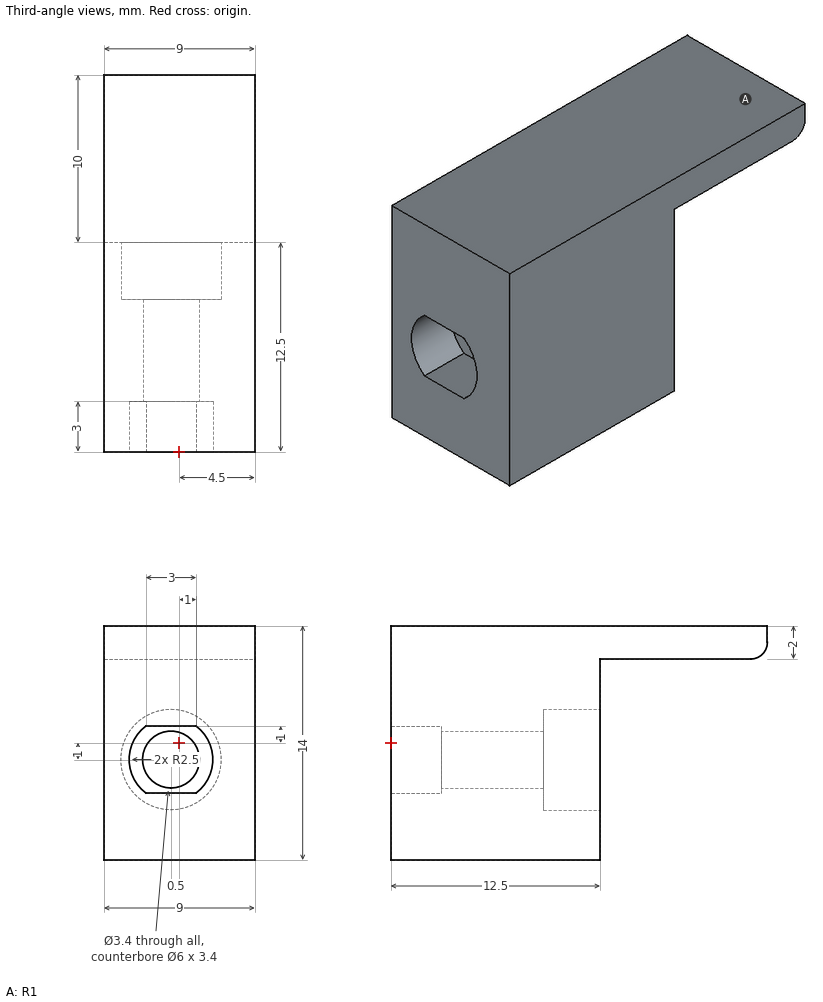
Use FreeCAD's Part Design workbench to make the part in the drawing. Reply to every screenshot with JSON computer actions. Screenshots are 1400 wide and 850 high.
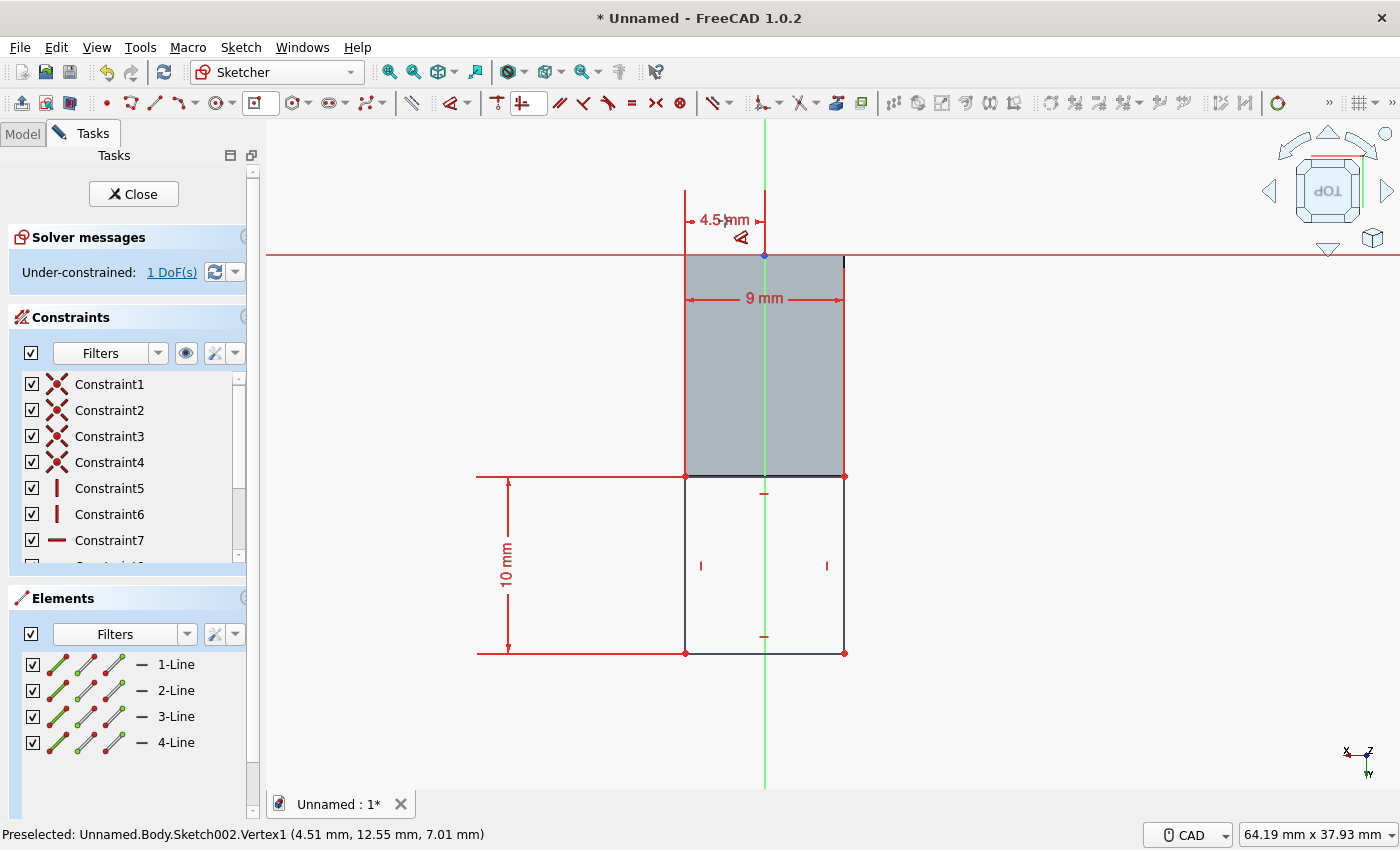
{"action": "left_click", "coordinate": [685, 477]}
{"action": "left_click", "coordinate": [651, 366]}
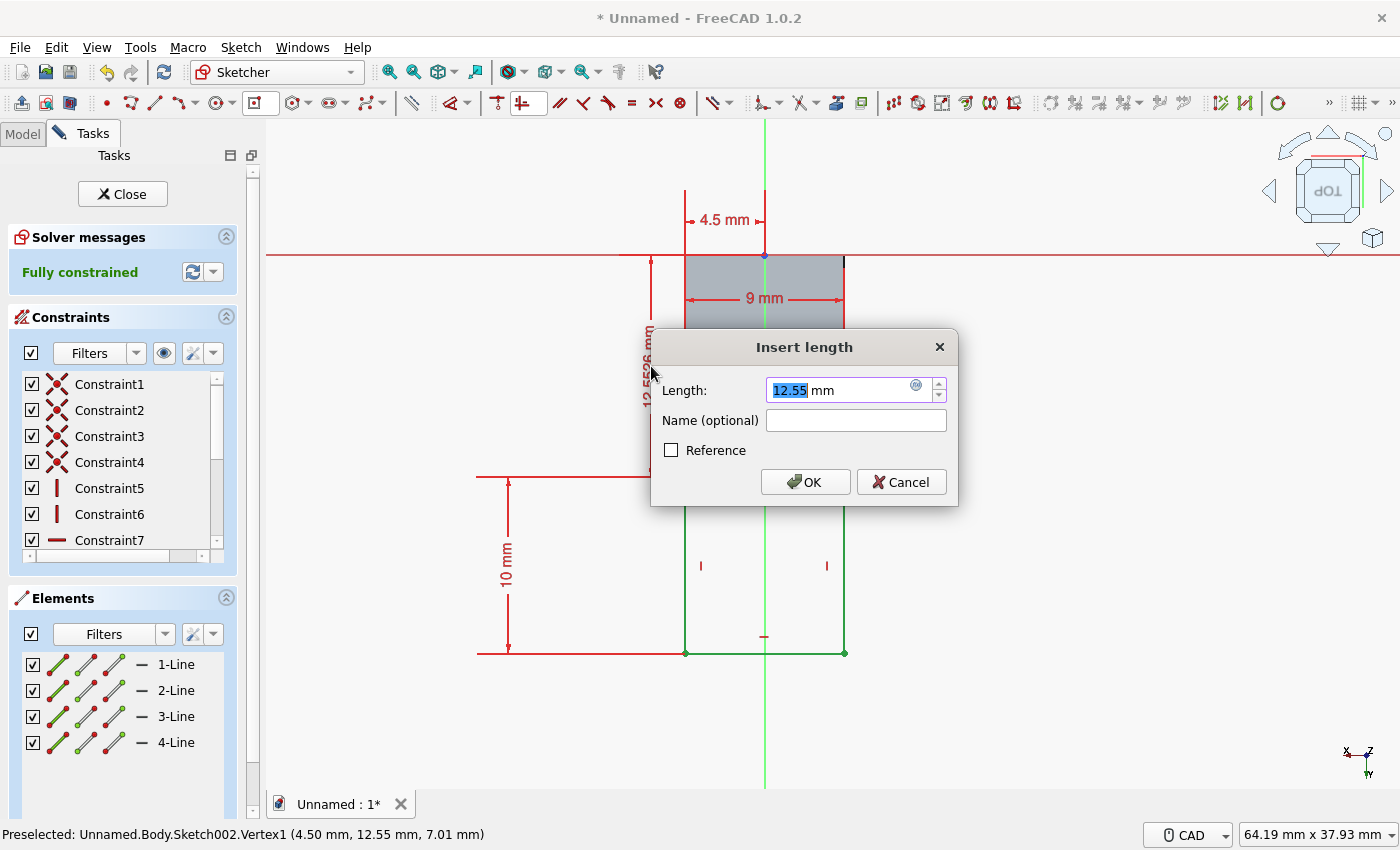
{"action": "type", "text": "12.5"}
{"action": "key", "text": "Return"}
{"action": "key", "text": "Escape"}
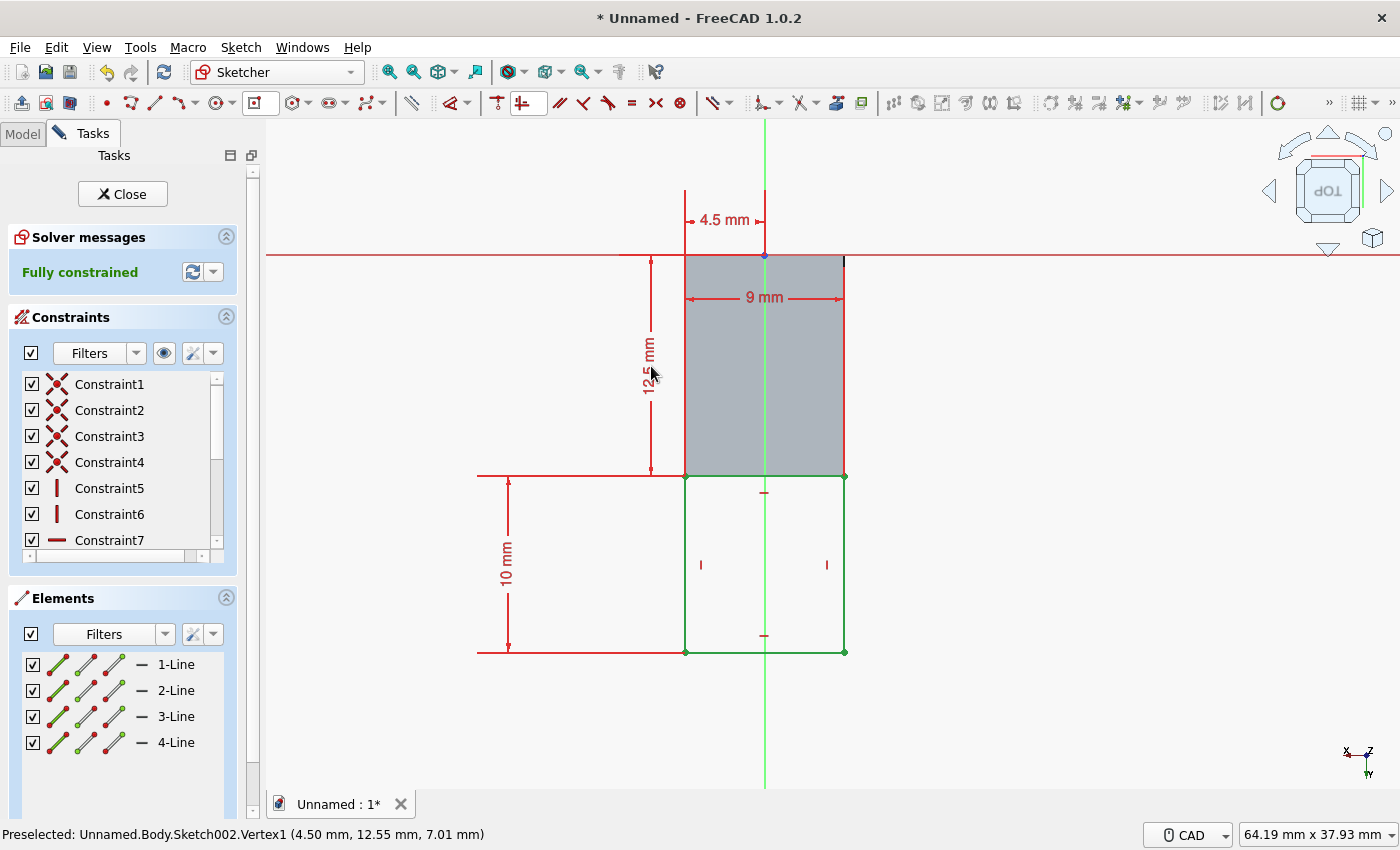
{"action": "left_click", "coordinate": [123, 194]}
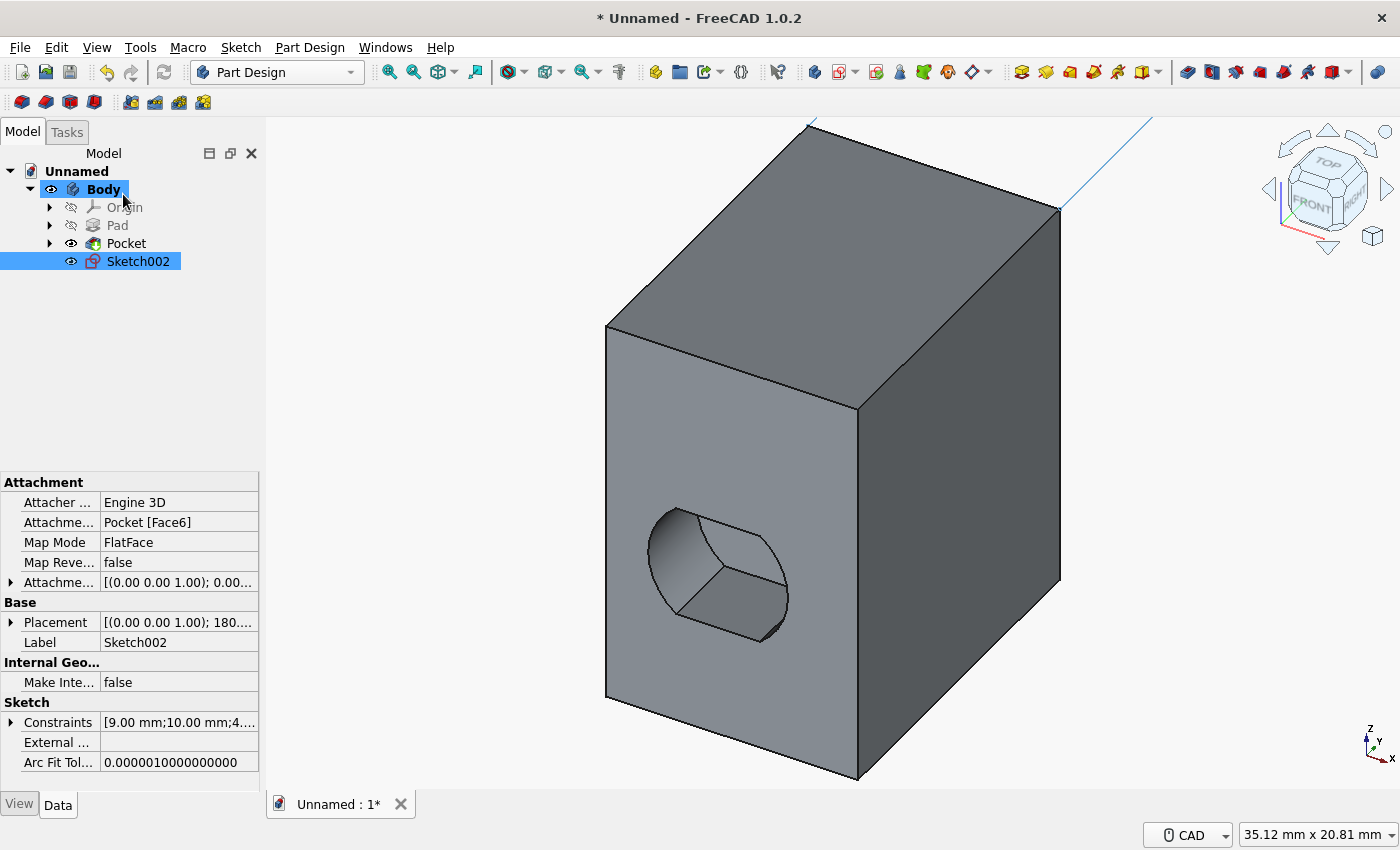
{"action": "left_click", "coordinate": [1022, 72]}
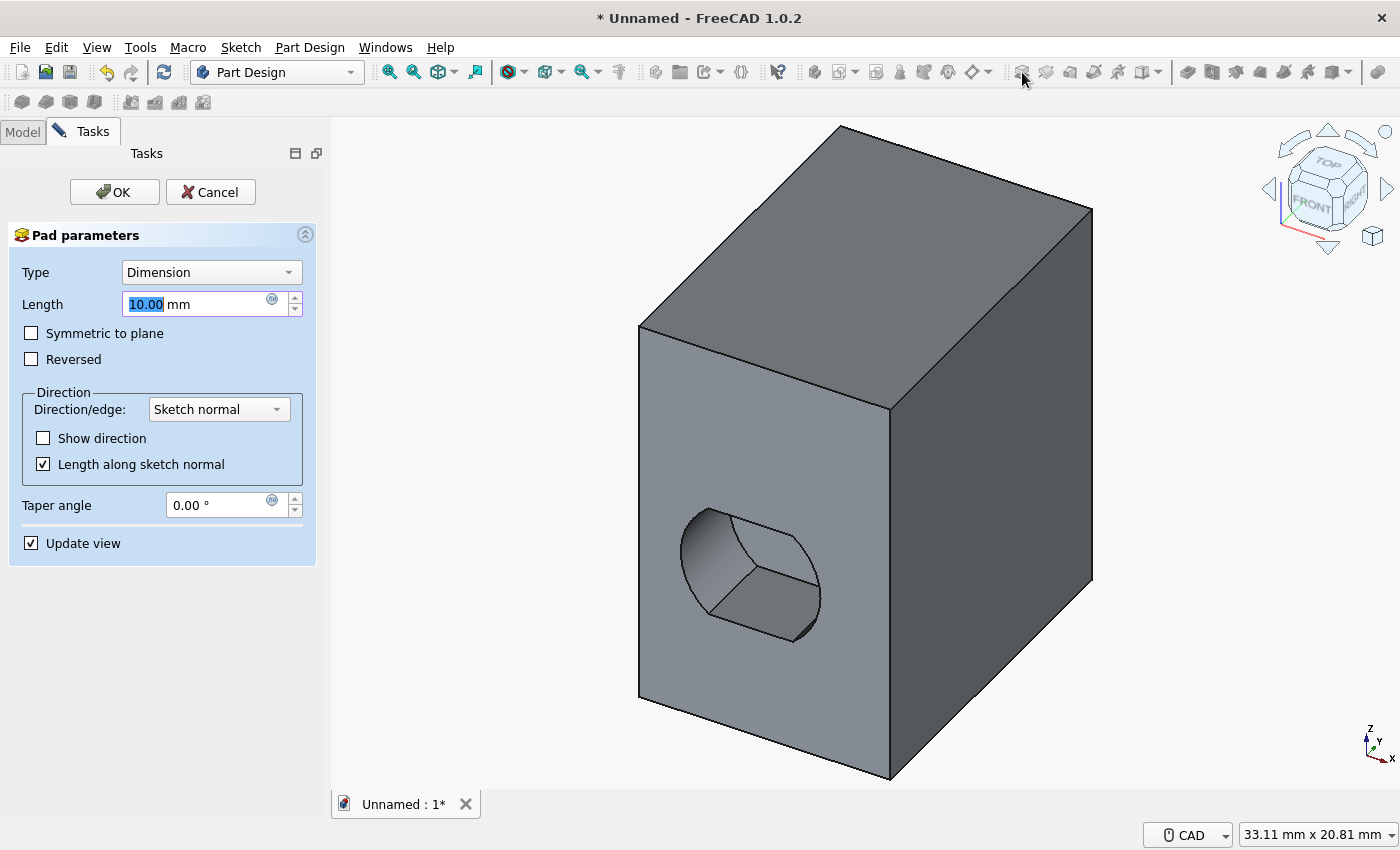
{"action": "type", "text": "2"}
{"action": "key", "text": "Tab"}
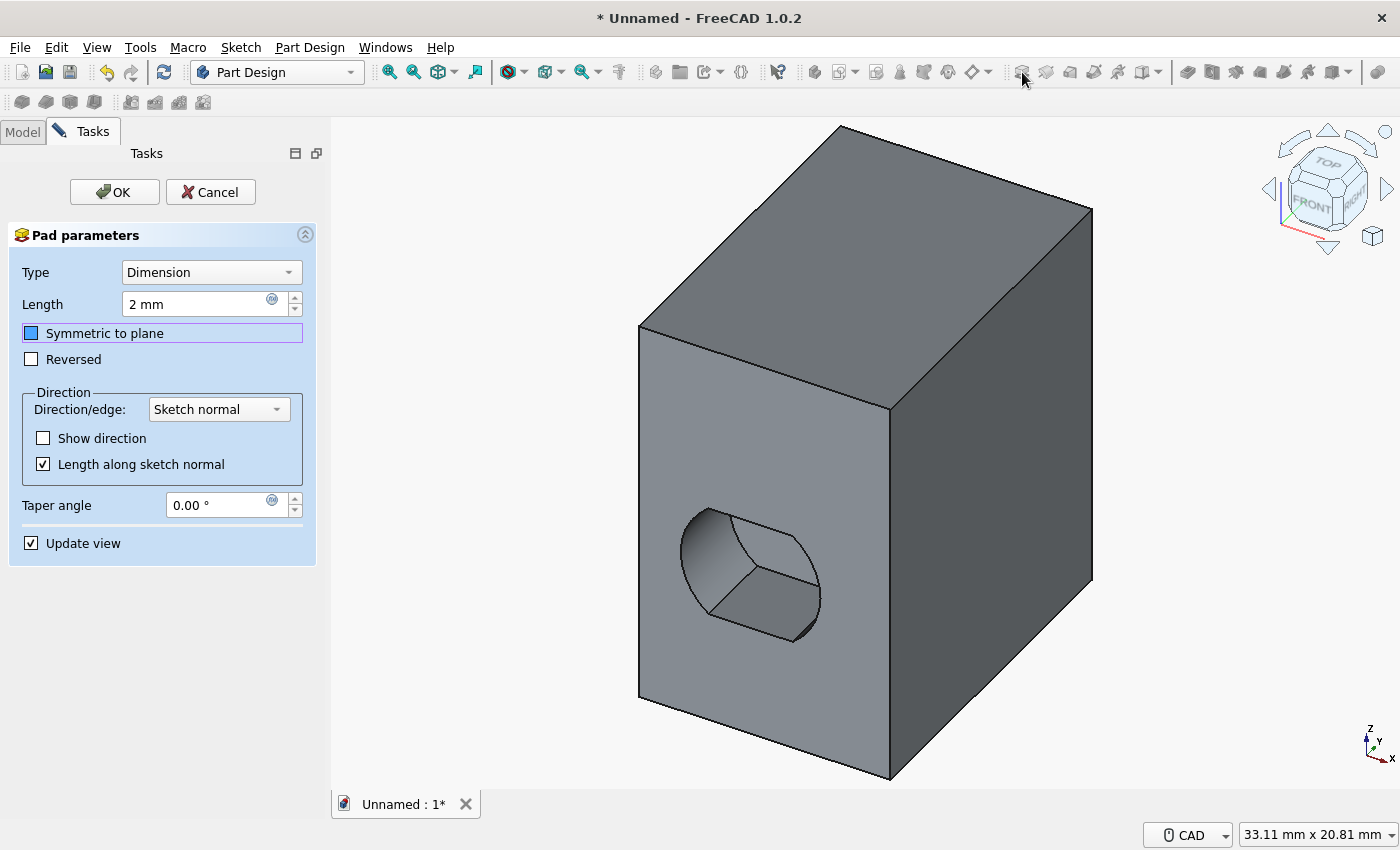
{"action": "left_click", "coordinate": [30, 359]}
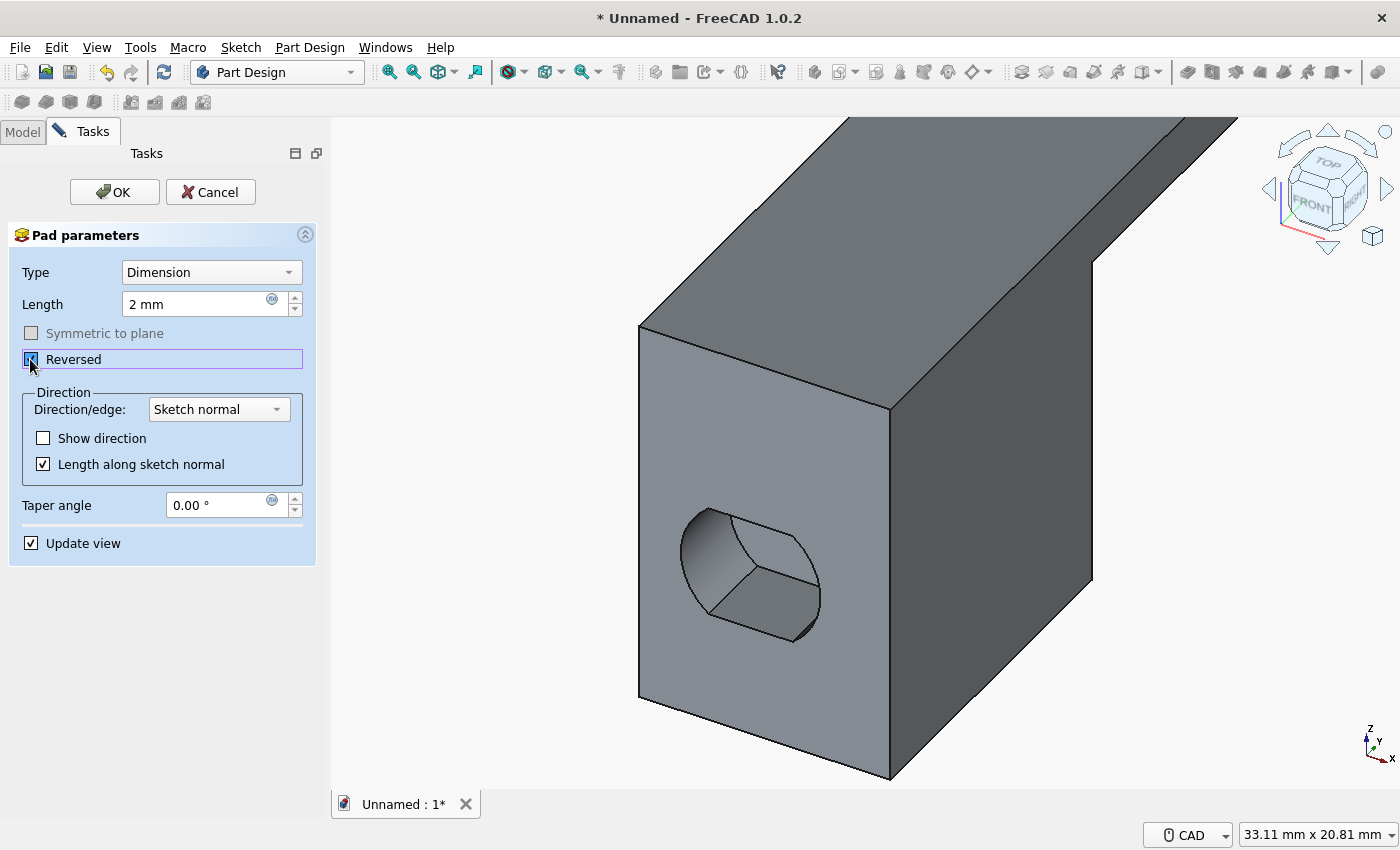
{"action": "left_click", "coordinate": [115, 192]}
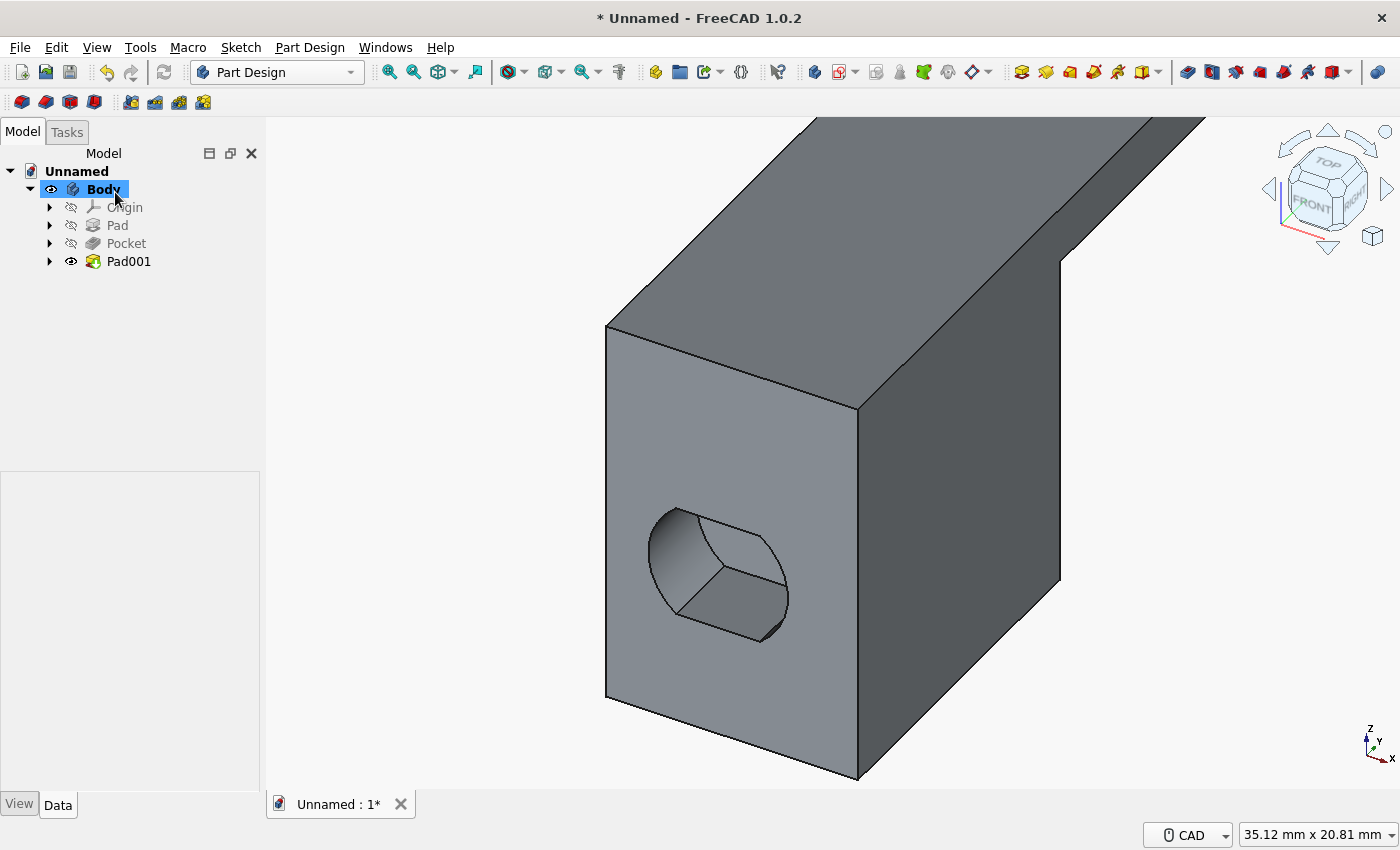
{"action": "key", "text": "v f"}